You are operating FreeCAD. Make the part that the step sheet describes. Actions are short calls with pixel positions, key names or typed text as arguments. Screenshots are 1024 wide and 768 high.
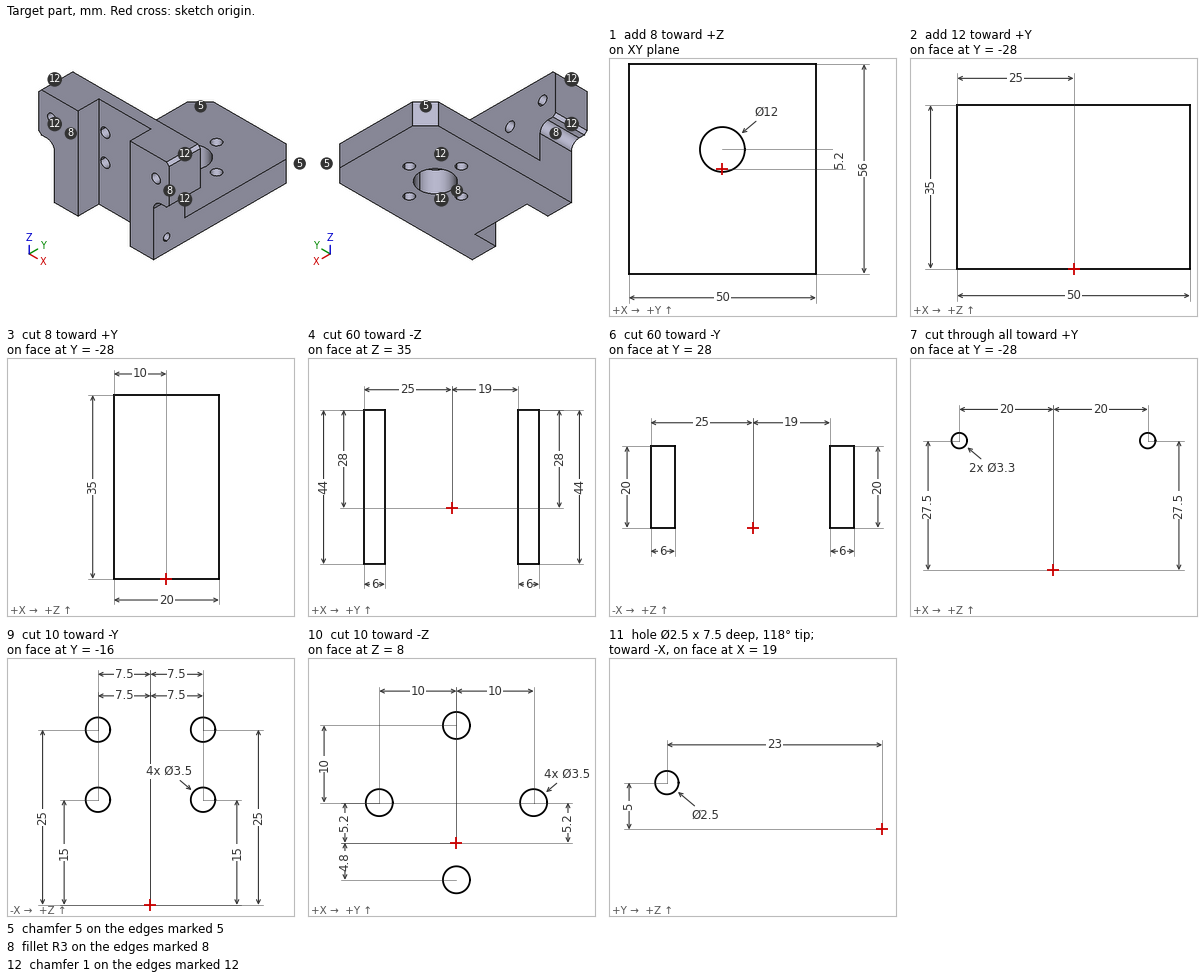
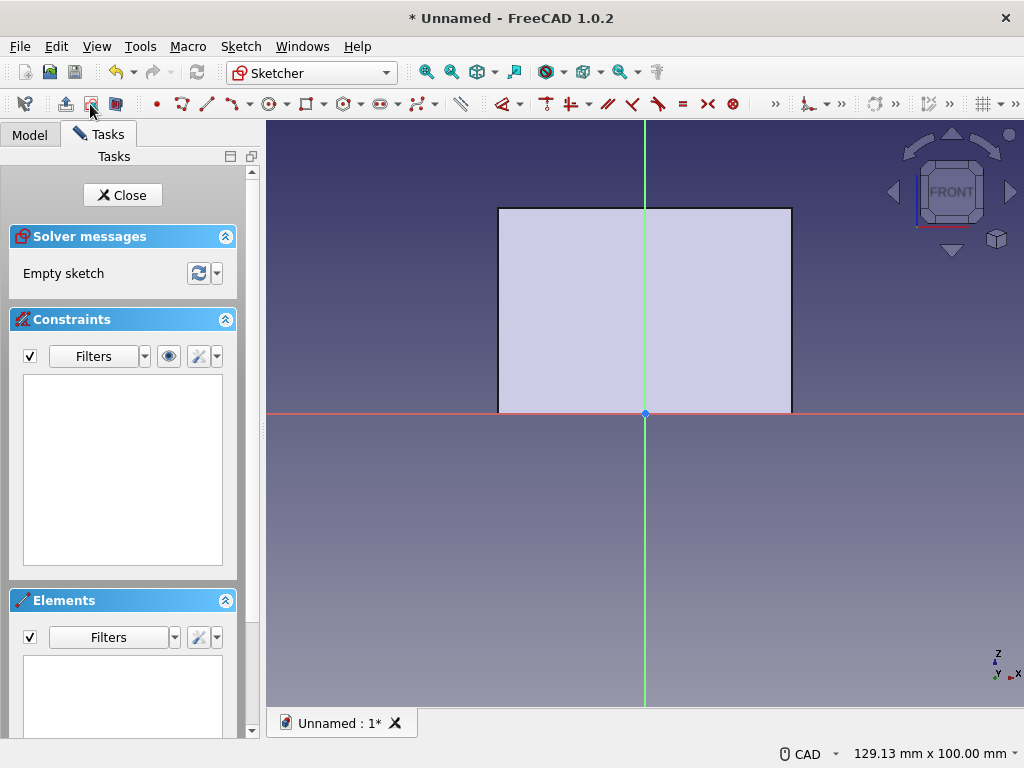
scroll(728, 186, up, 3)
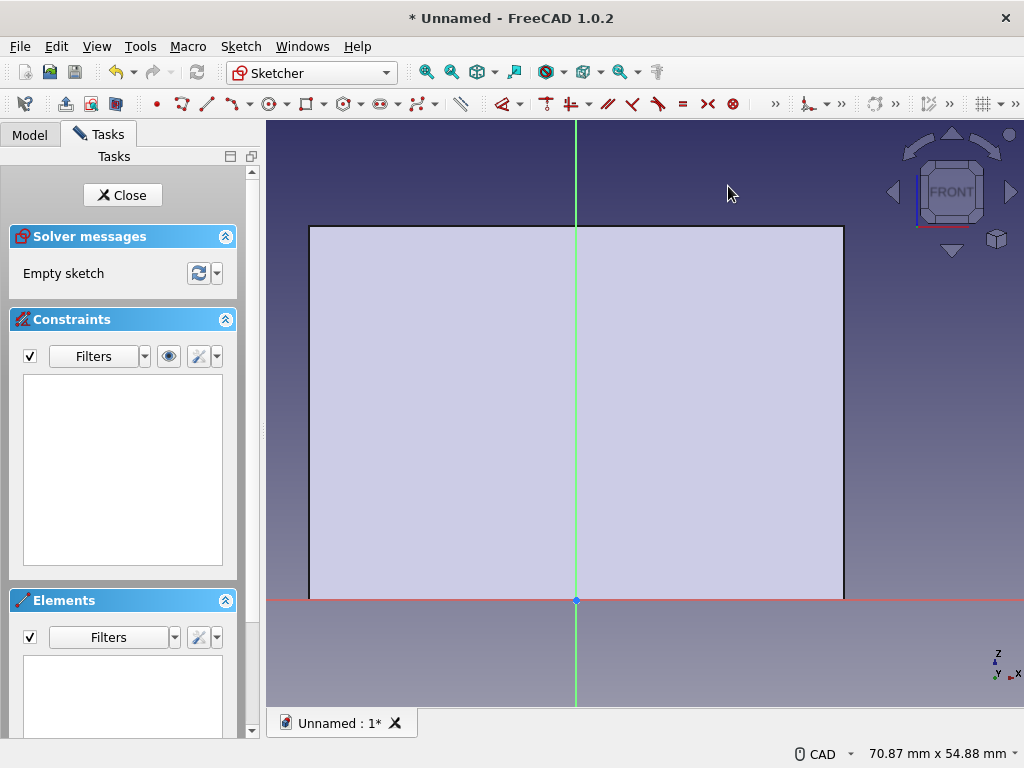
click(306, 104)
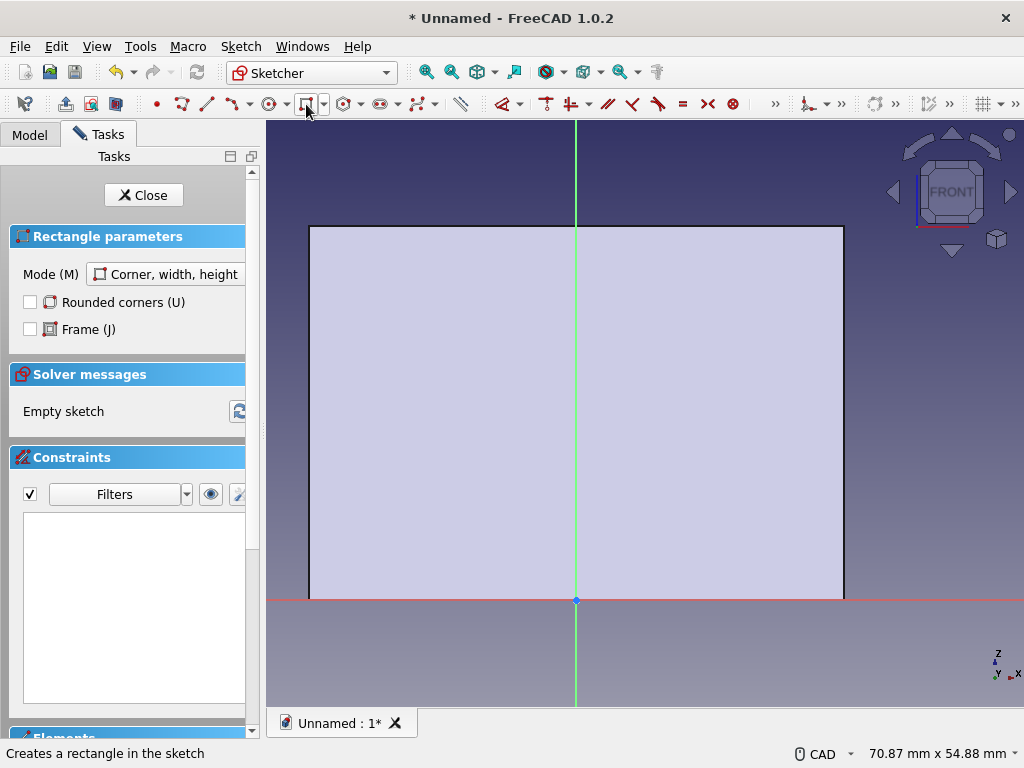
click(469, 226)
click(683, 600)
key(Escape)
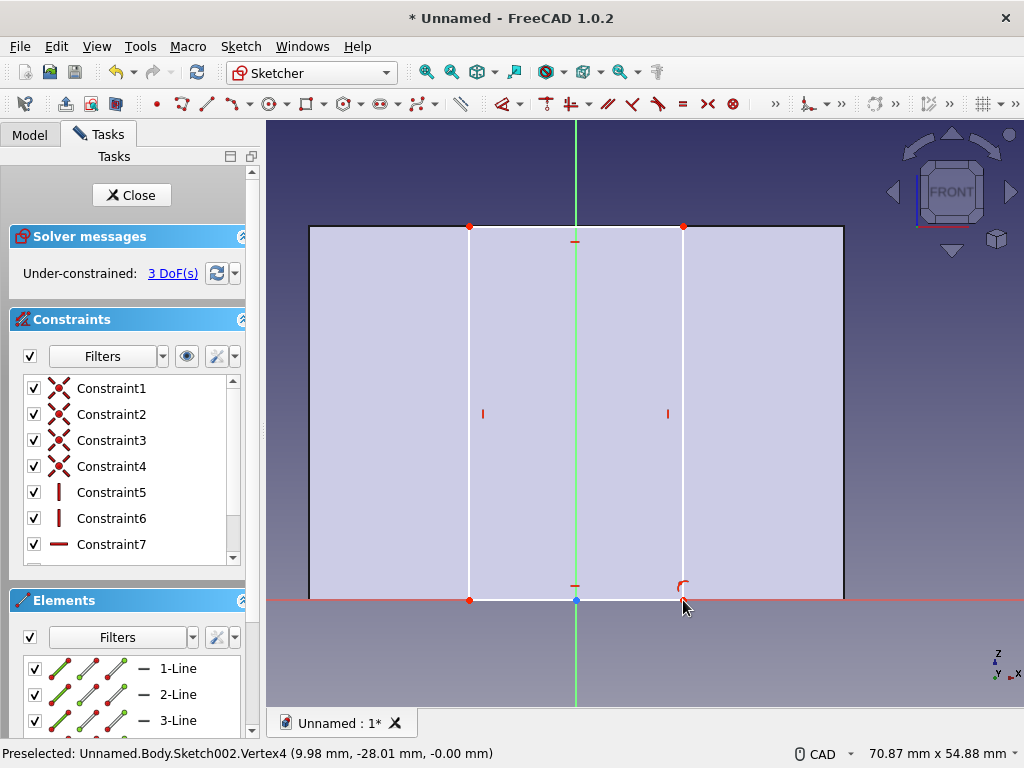
click(502, 104)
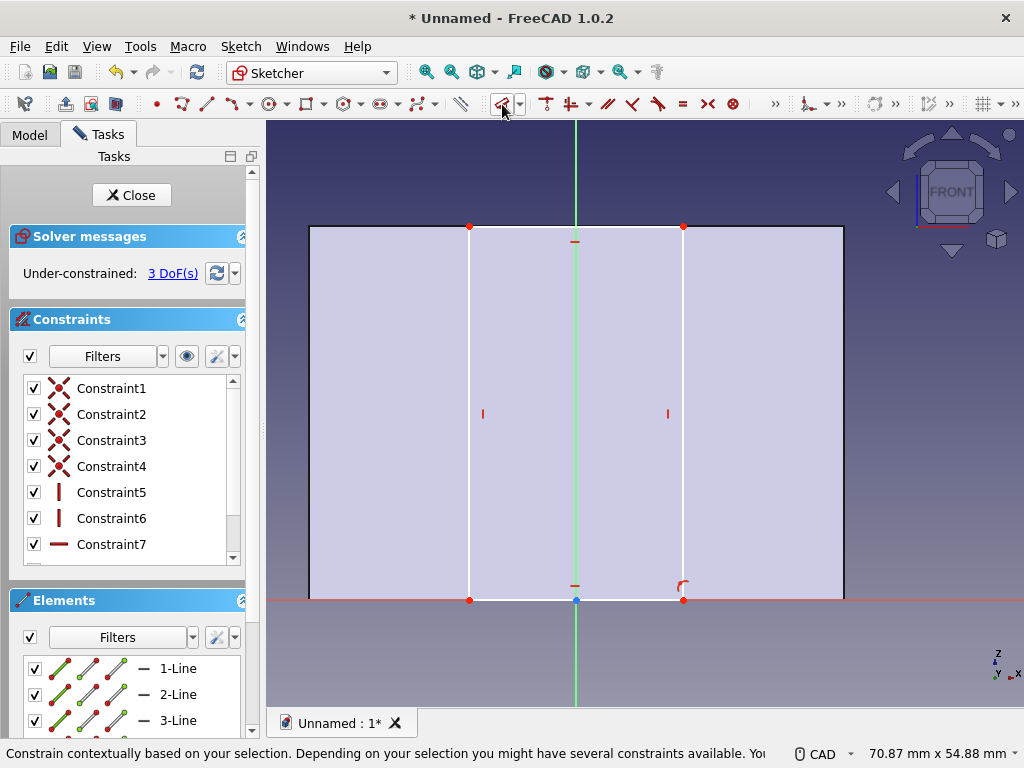
click(469, 339)
click(435, 414)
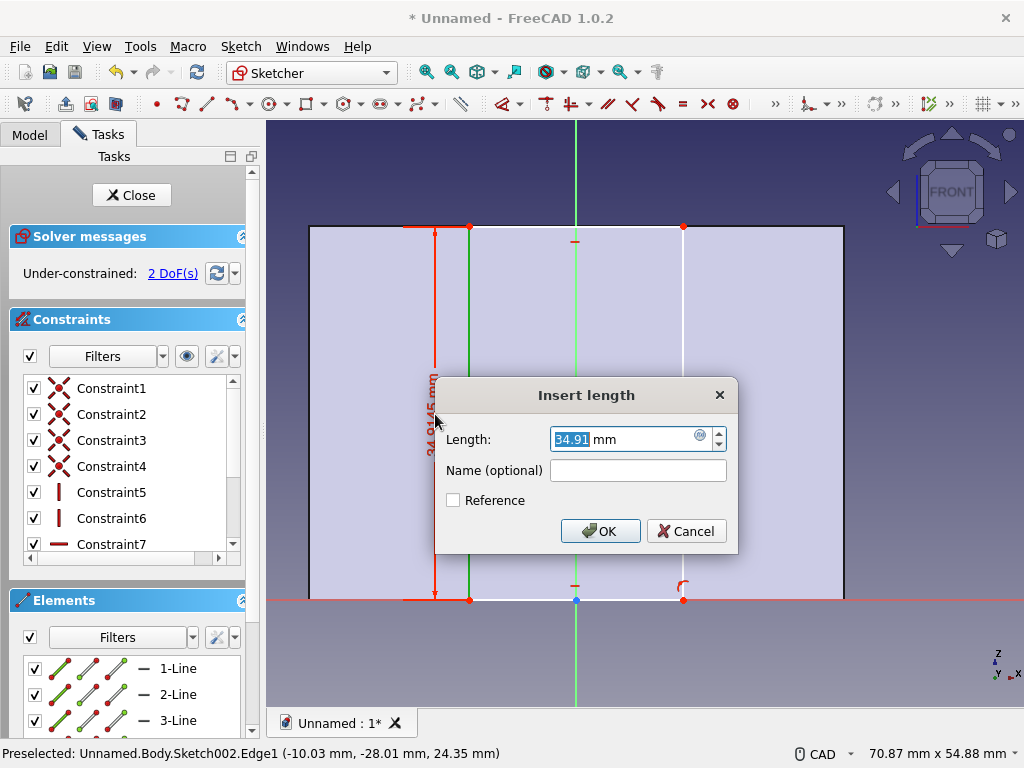
text(35)
key(Return)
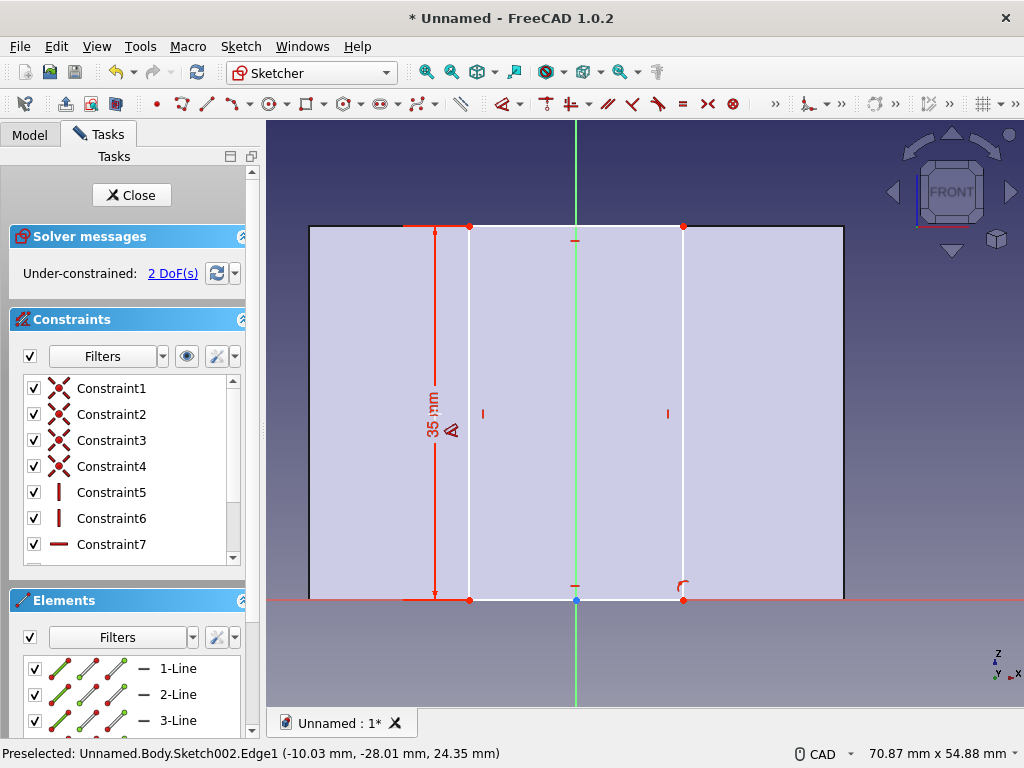
click(533, 600)
click(527, 634)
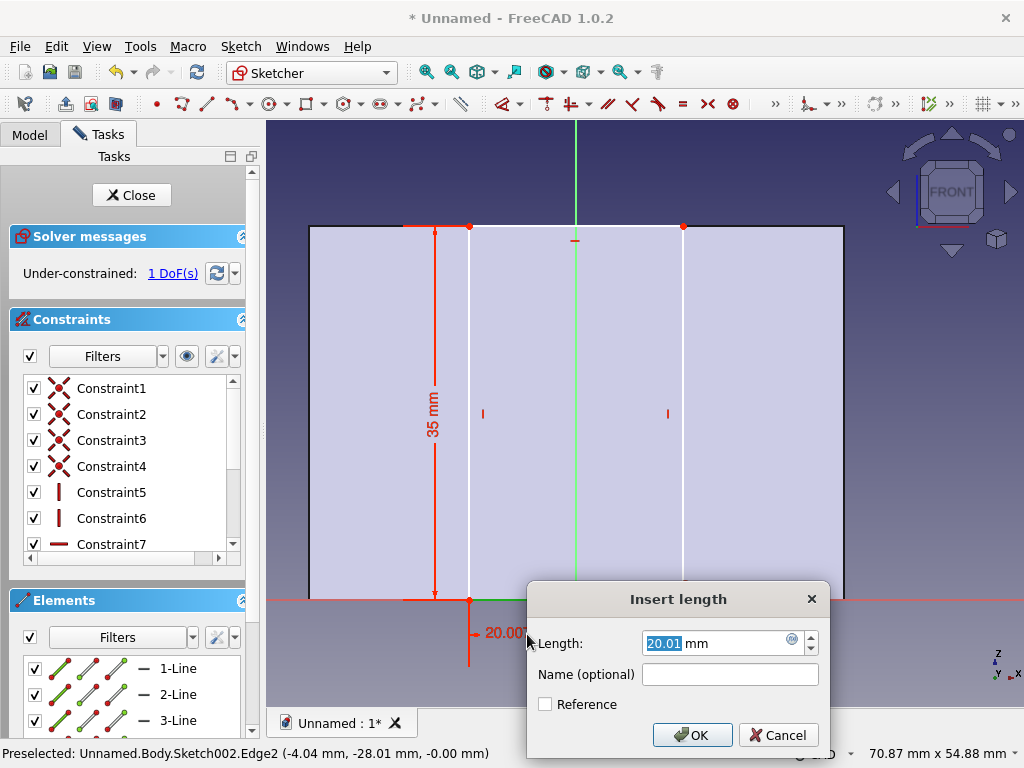
text(20)
key(Return)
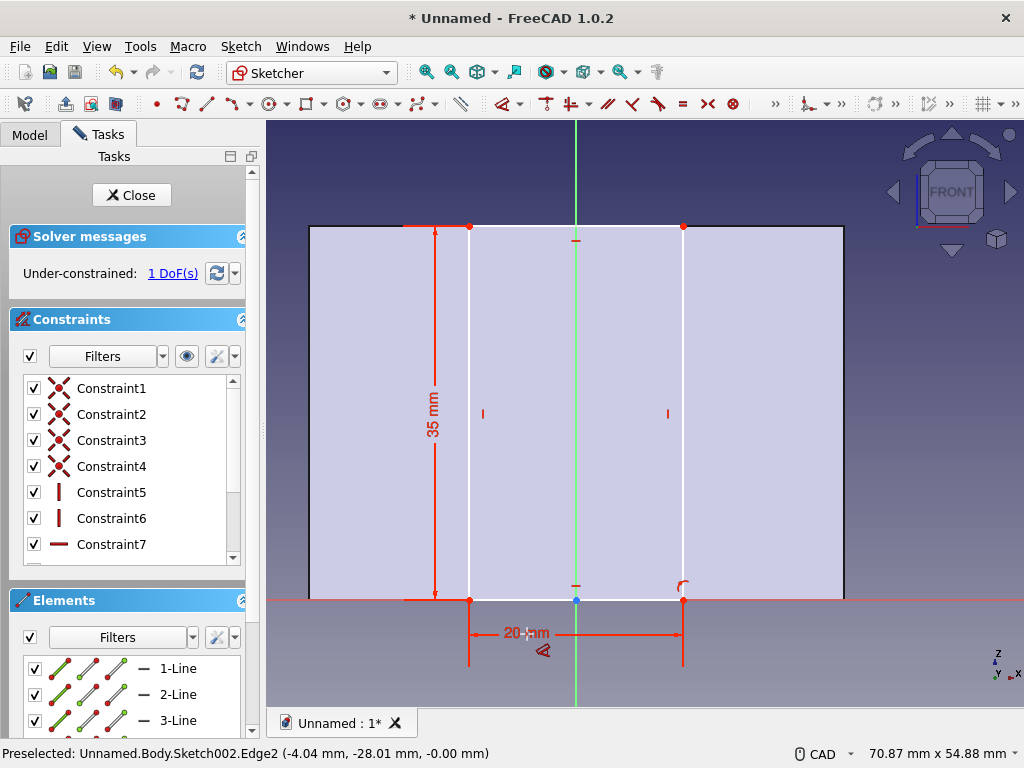
click(469, 226)
click(523, 192)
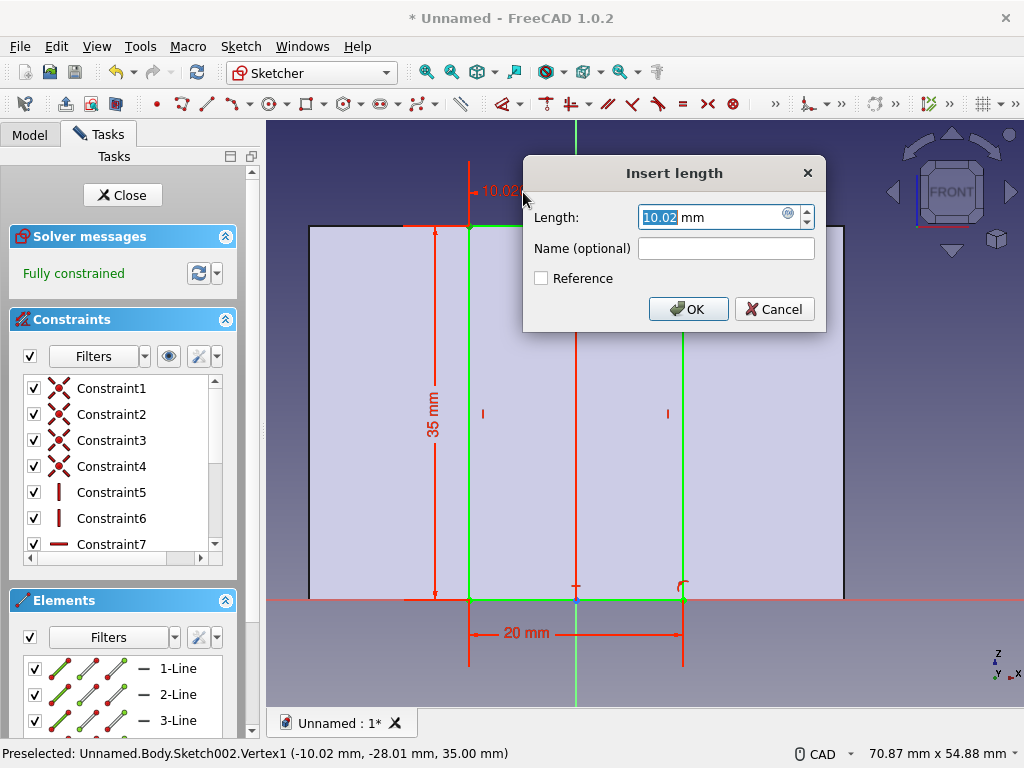
text(10)
key(Return)
key(Escape)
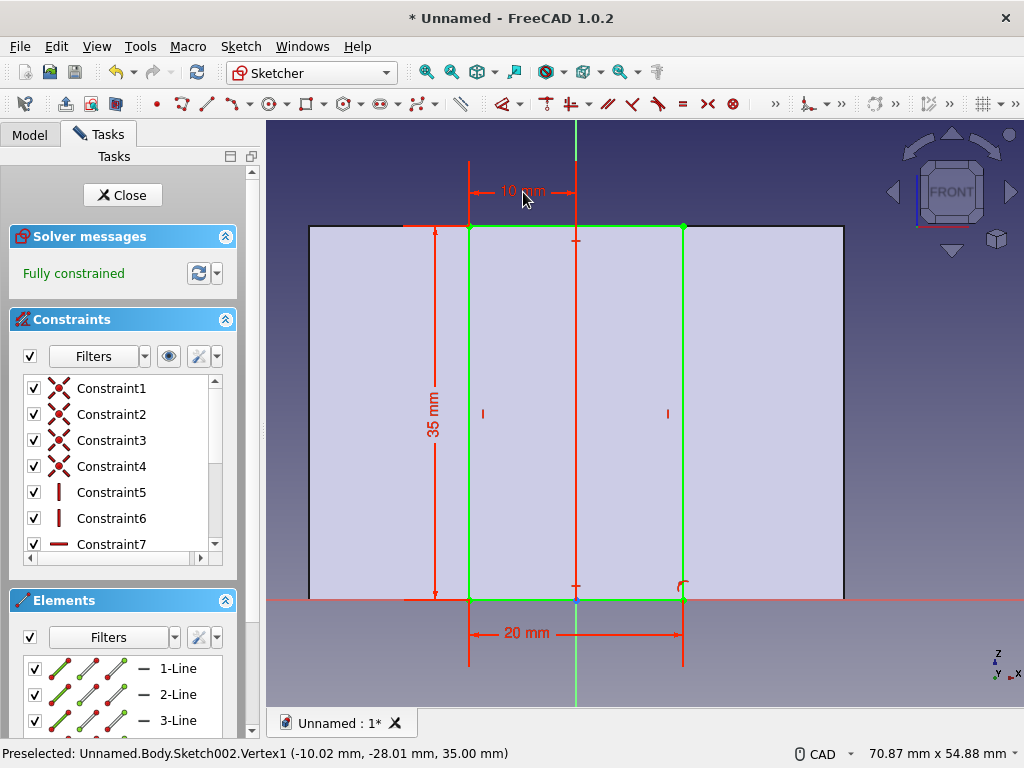
click(123, 195)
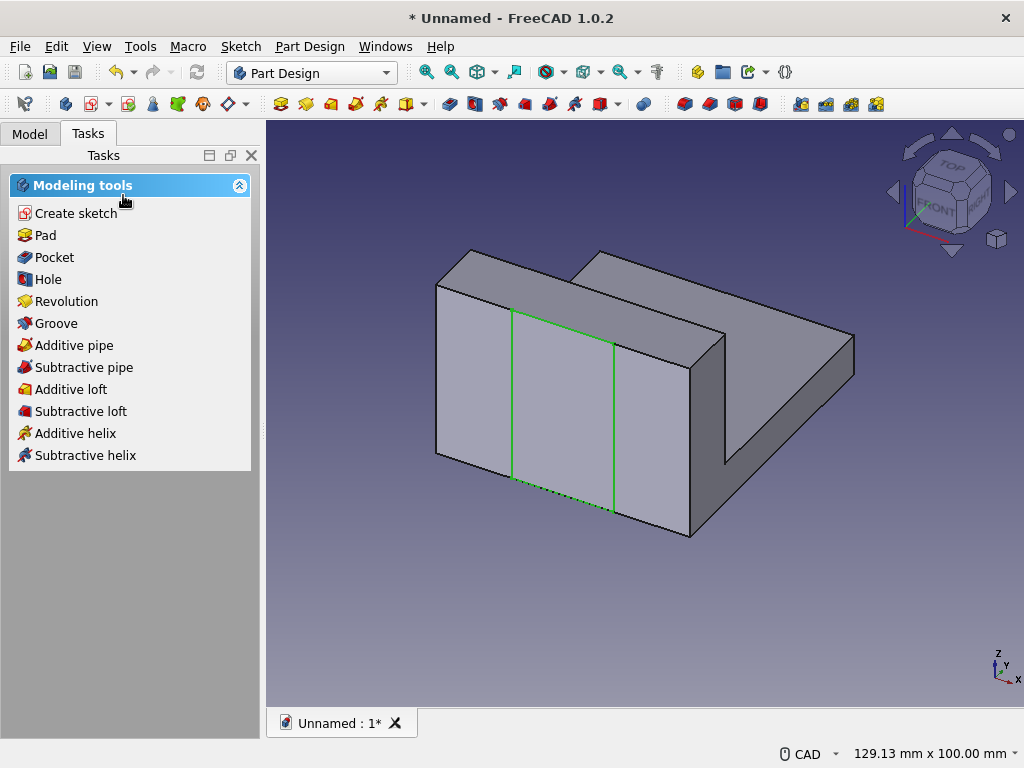
click(450, 104)